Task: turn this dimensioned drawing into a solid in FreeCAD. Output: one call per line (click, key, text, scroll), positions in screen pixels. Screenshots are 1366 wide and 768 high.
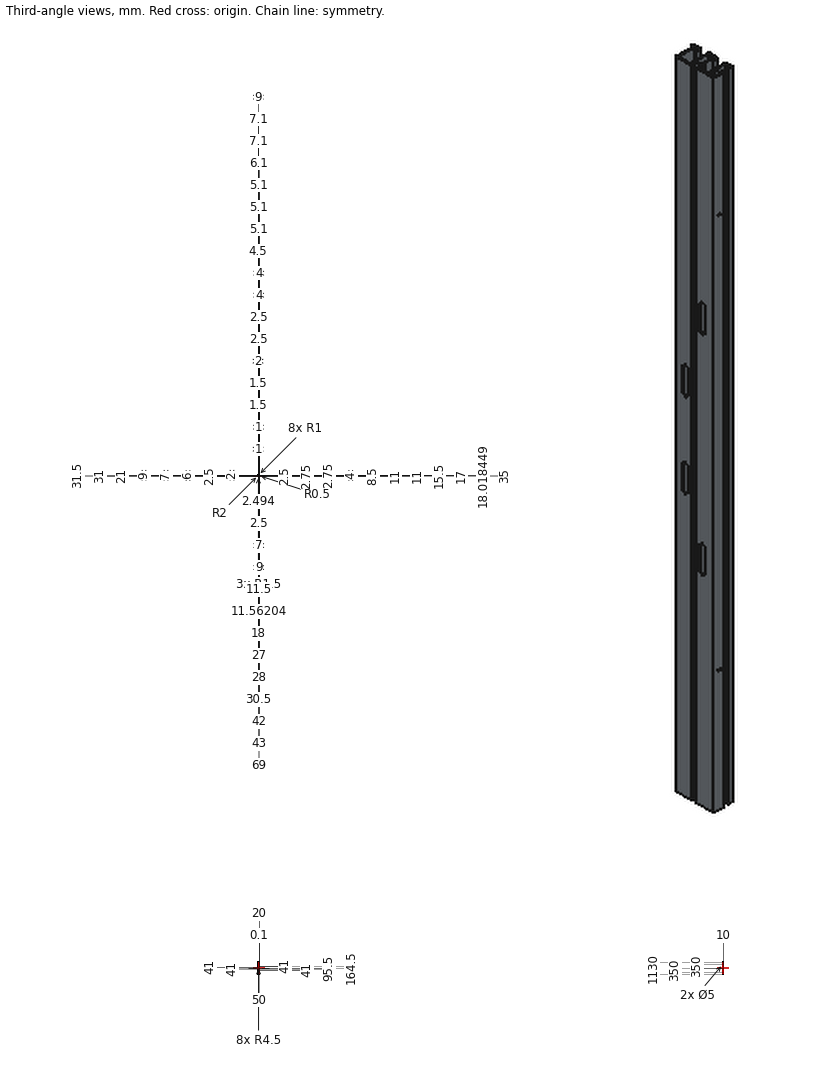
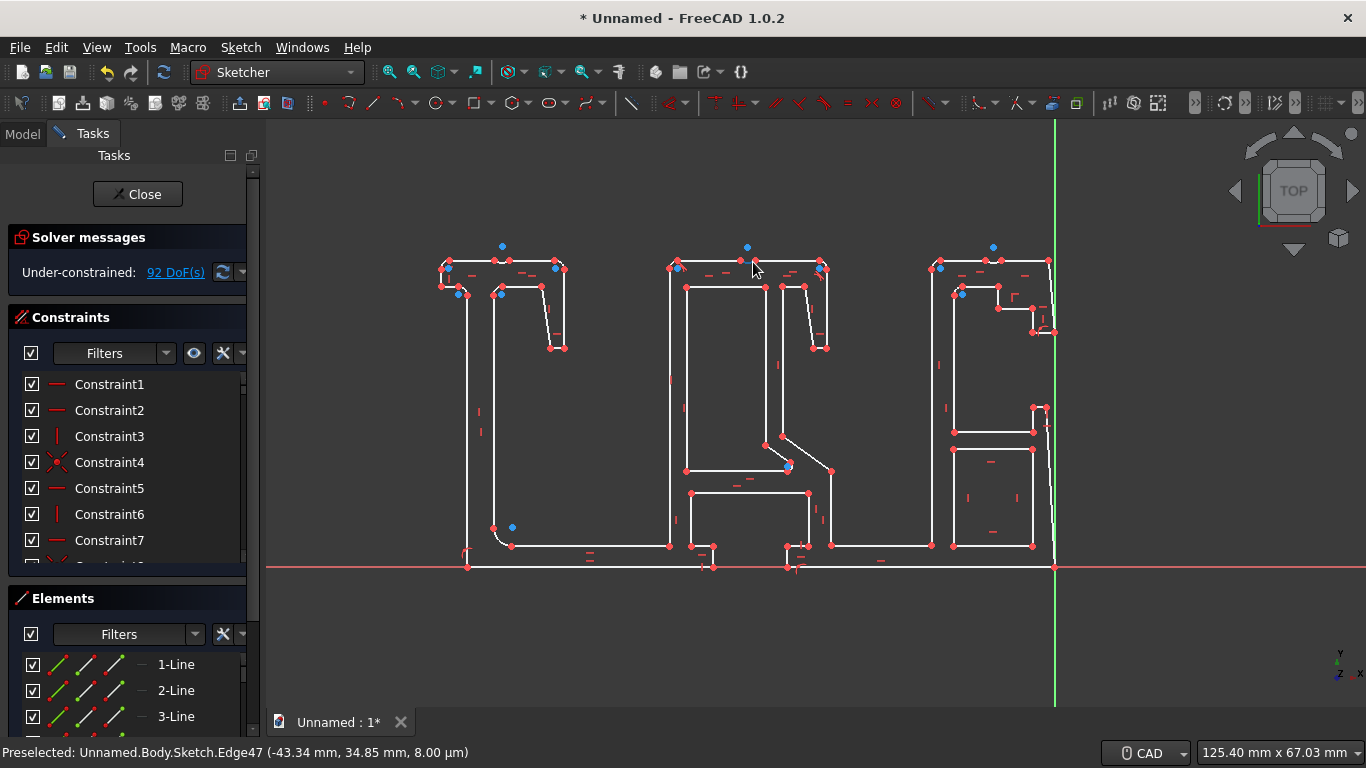
click(622, 546)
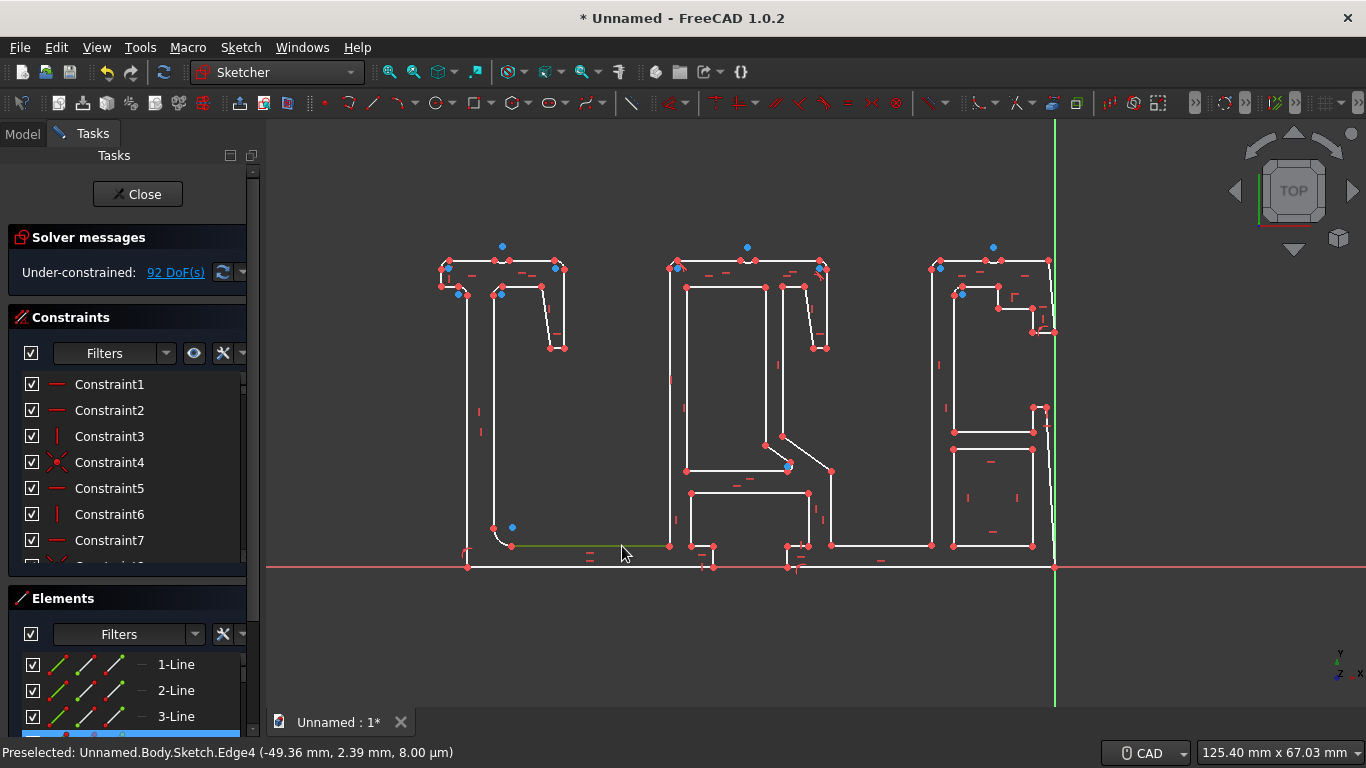
click(499, 540)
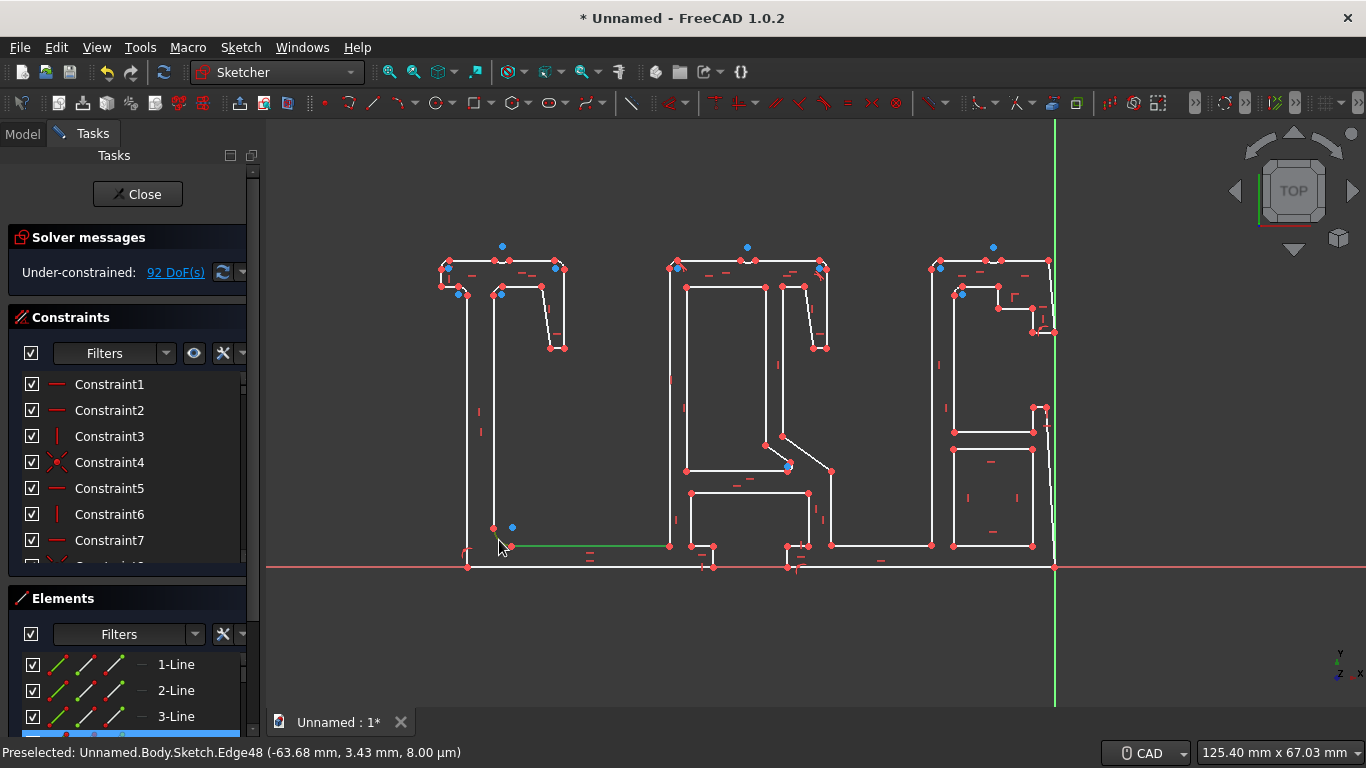
key(t)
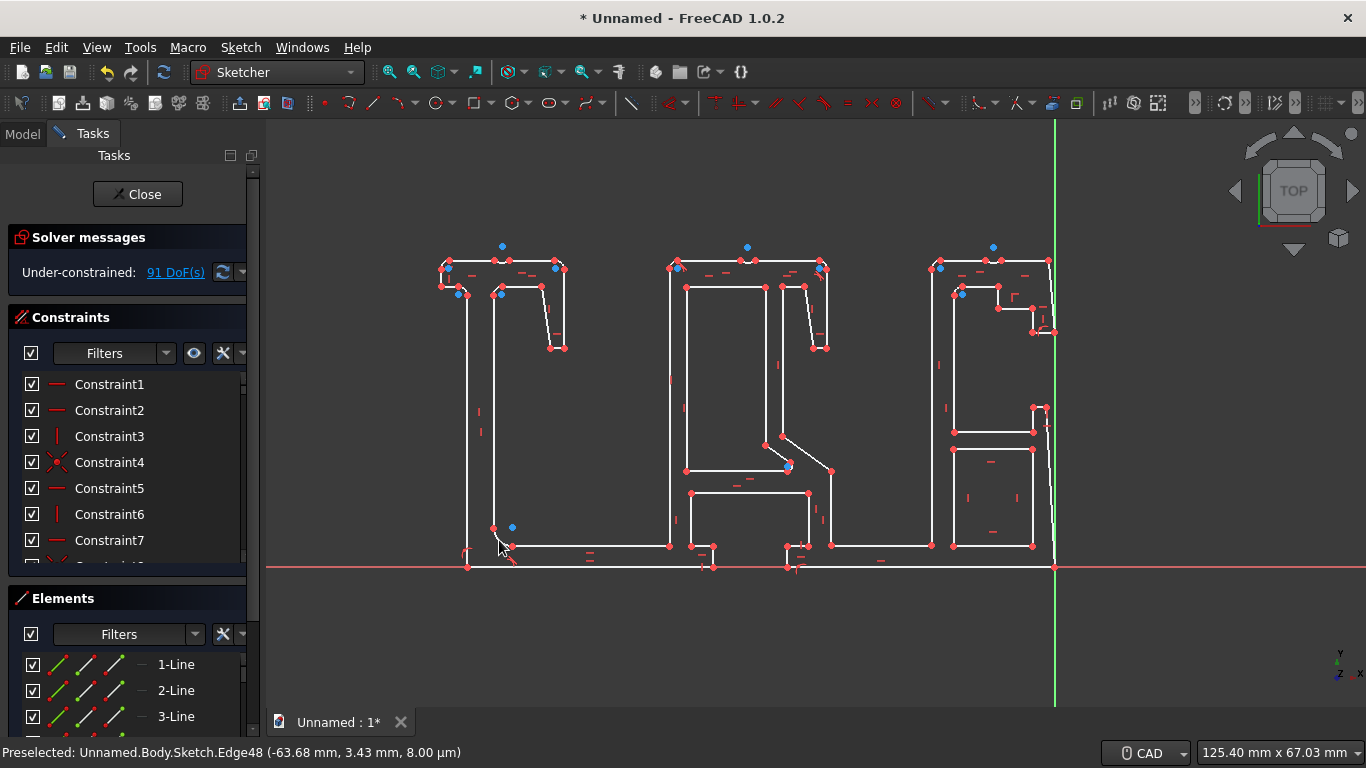
click(494, 458)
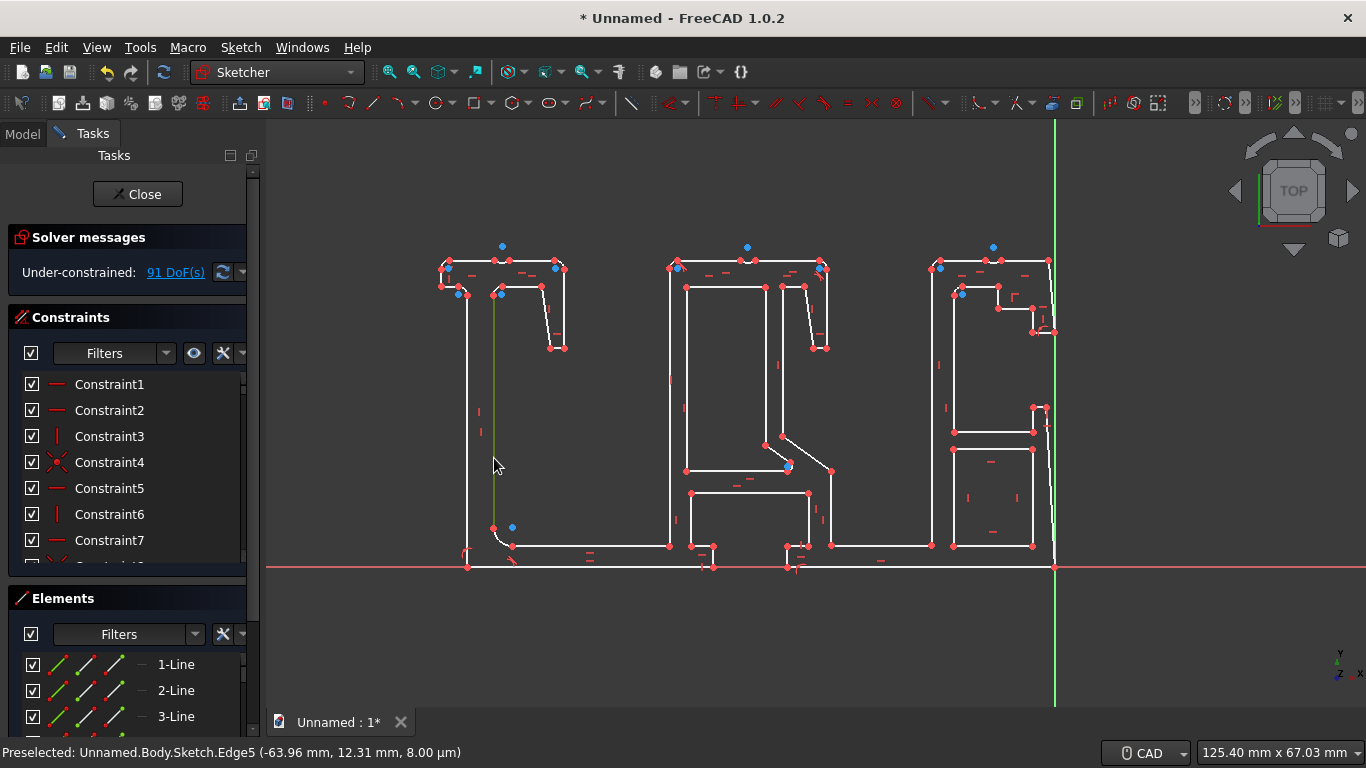
click(499, 541)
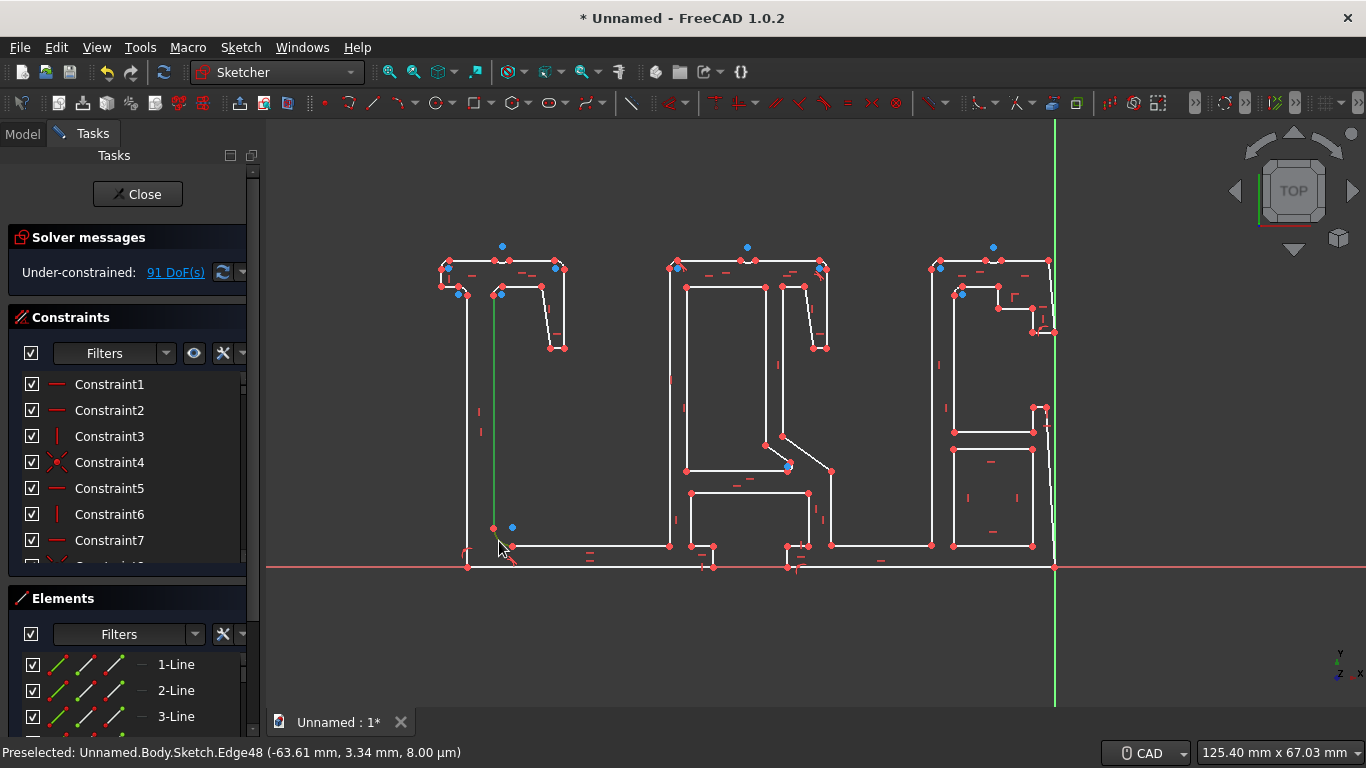
click(824, 104)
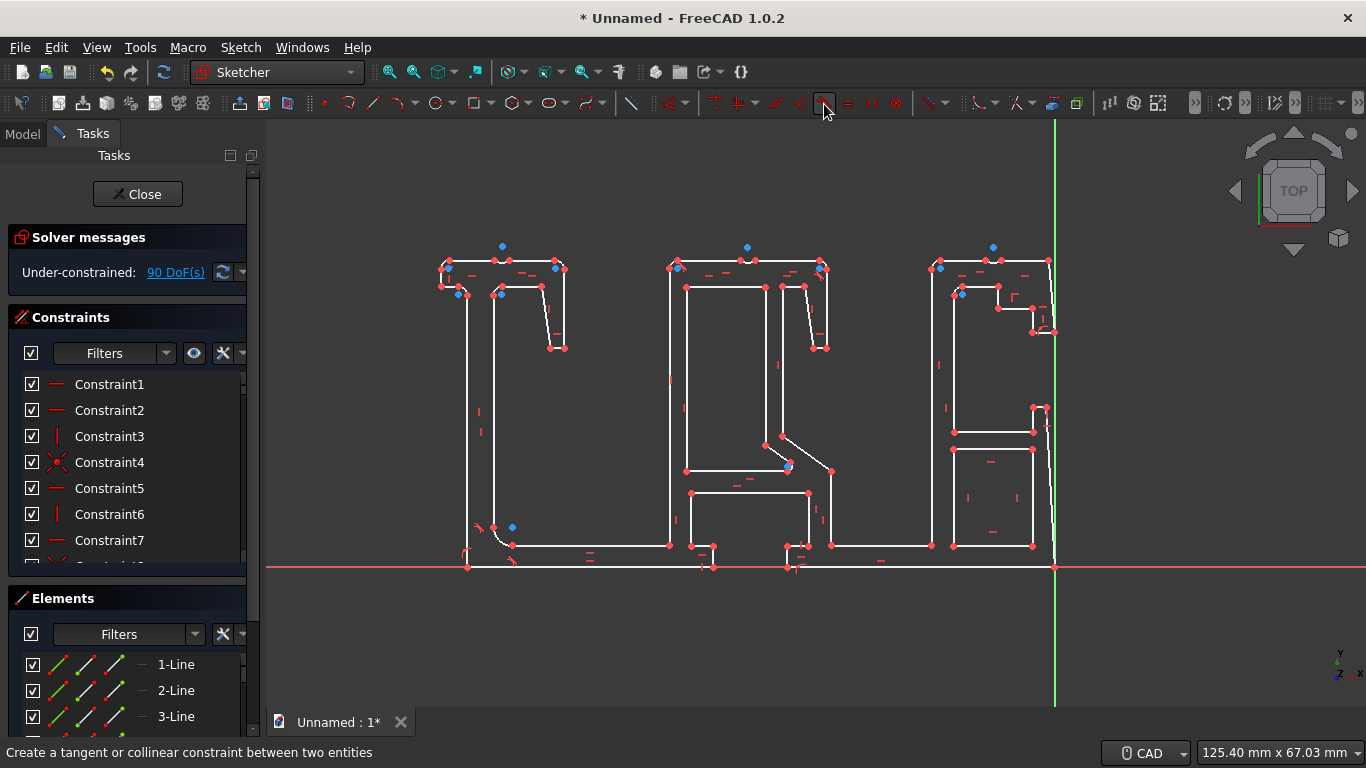
click(494, 458)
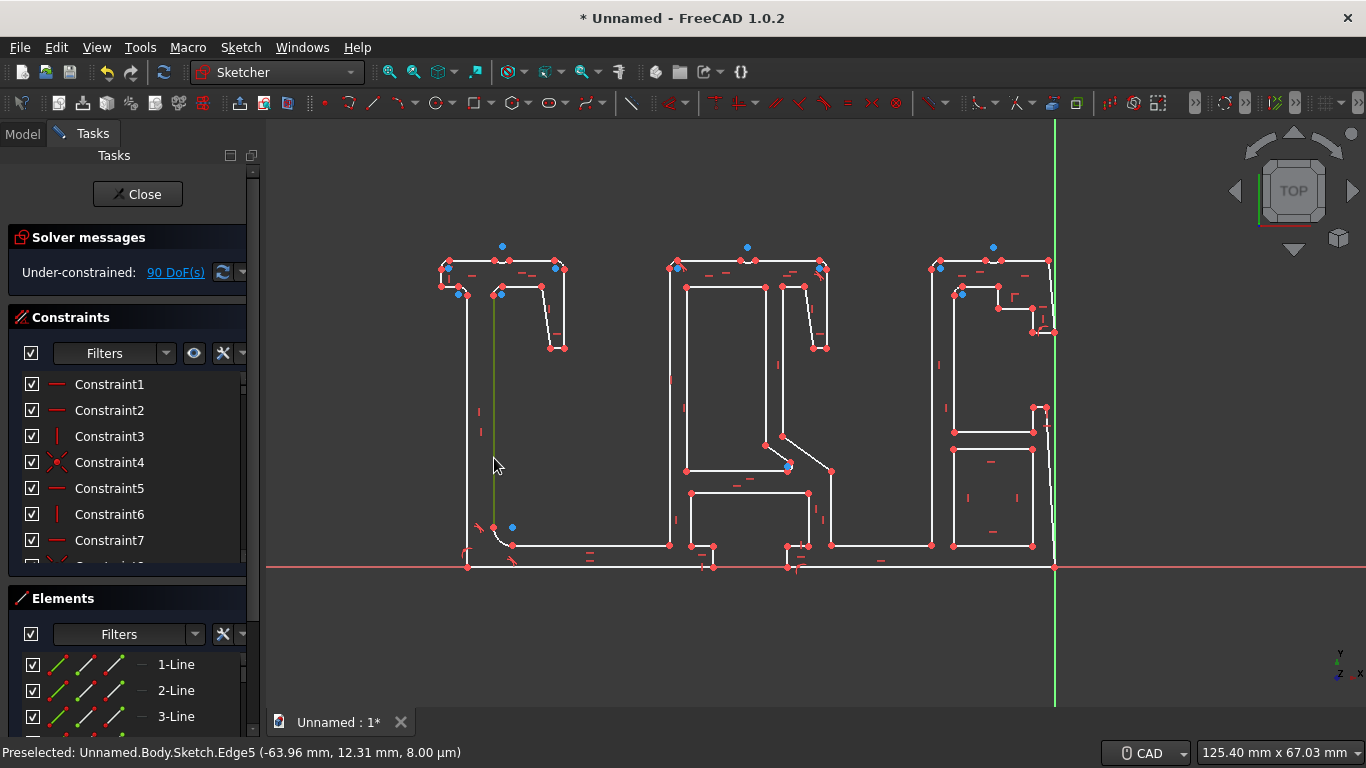
scroll(496, 289, up, 4)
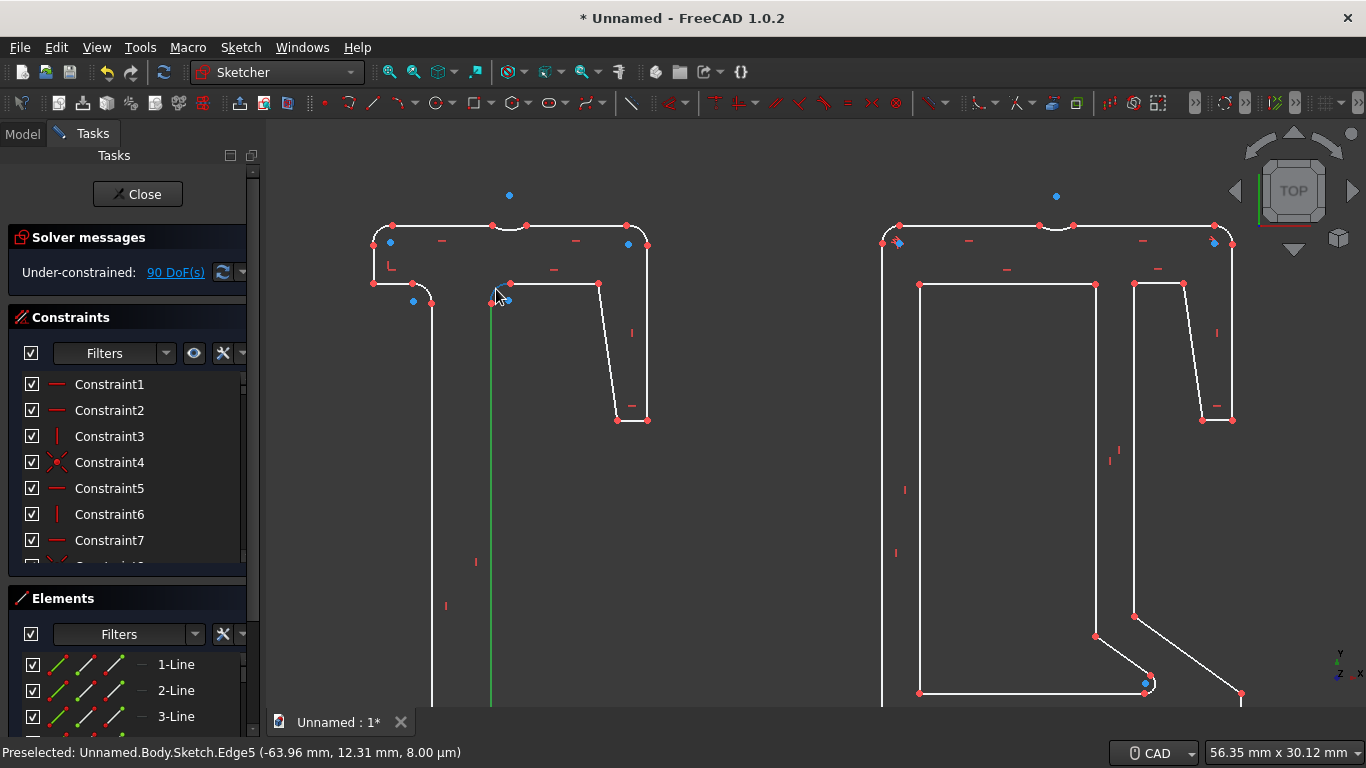
click(496, 289)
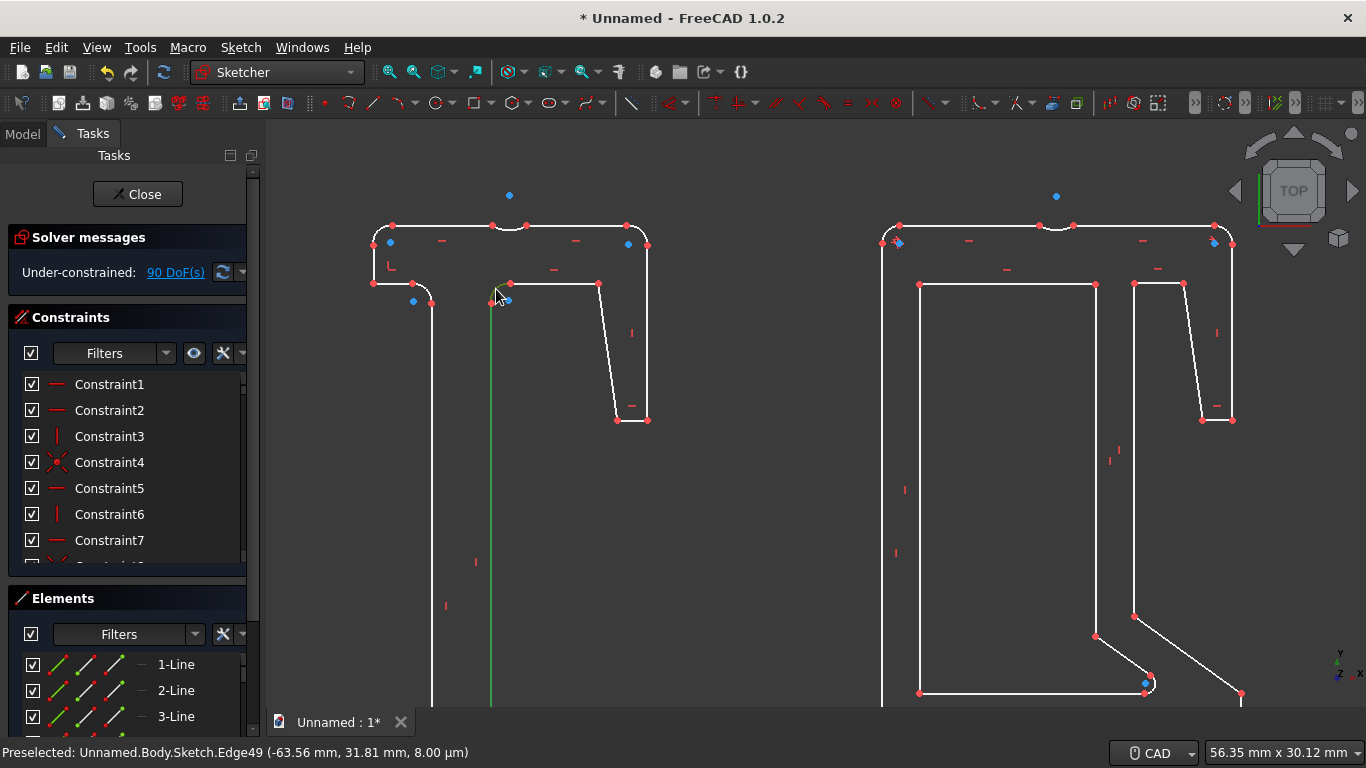
click(824, 104)